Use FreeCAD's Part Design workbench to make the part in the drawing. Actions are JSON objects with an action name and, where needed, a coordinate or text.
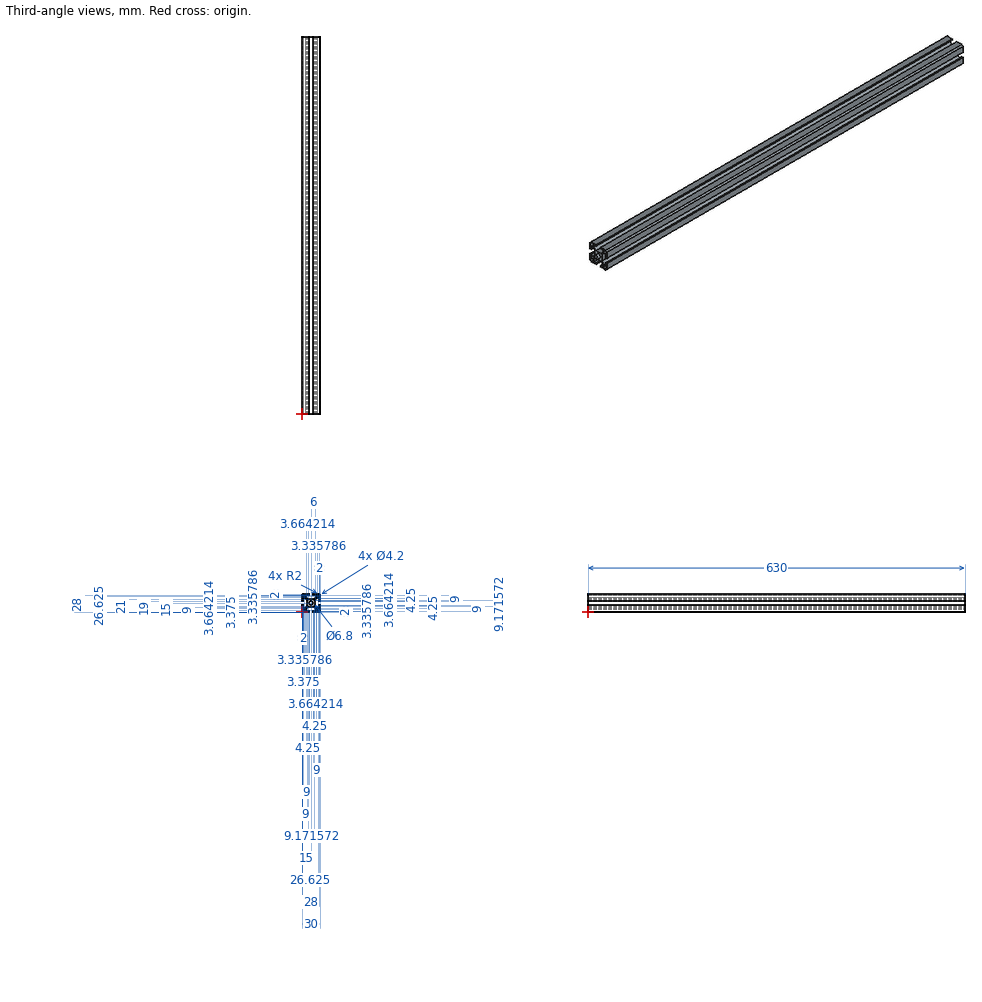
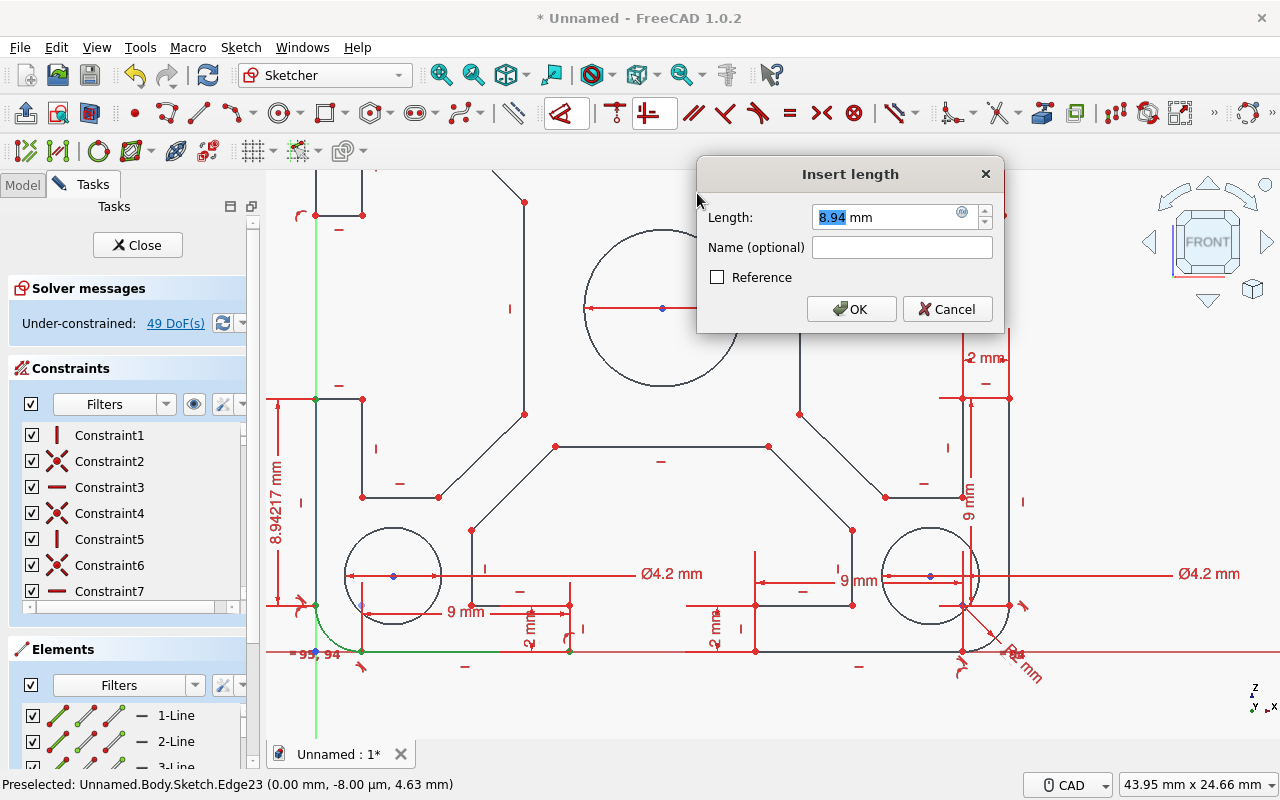
{"action": "type", "text": "9"}
{"action": "key", "text": "Return"}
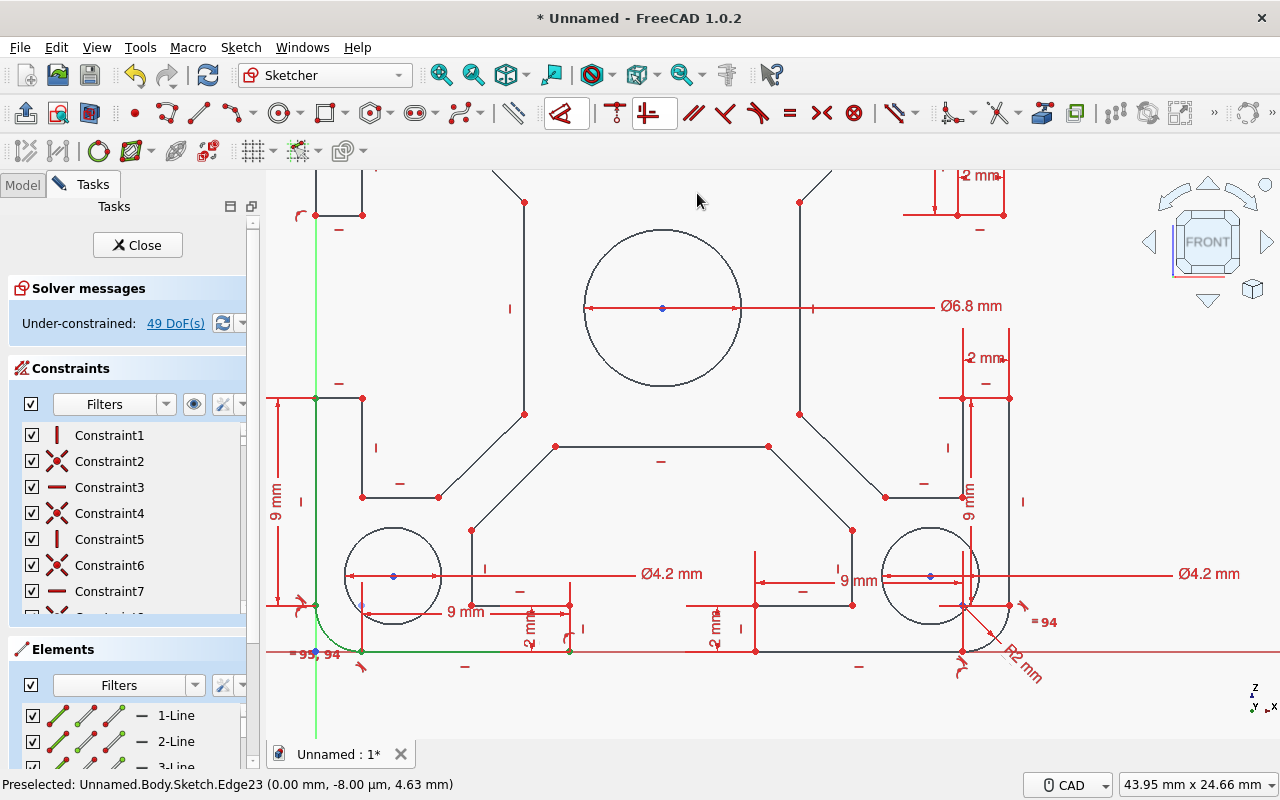
{"action": "left_click", "coordinate": [330, 398]}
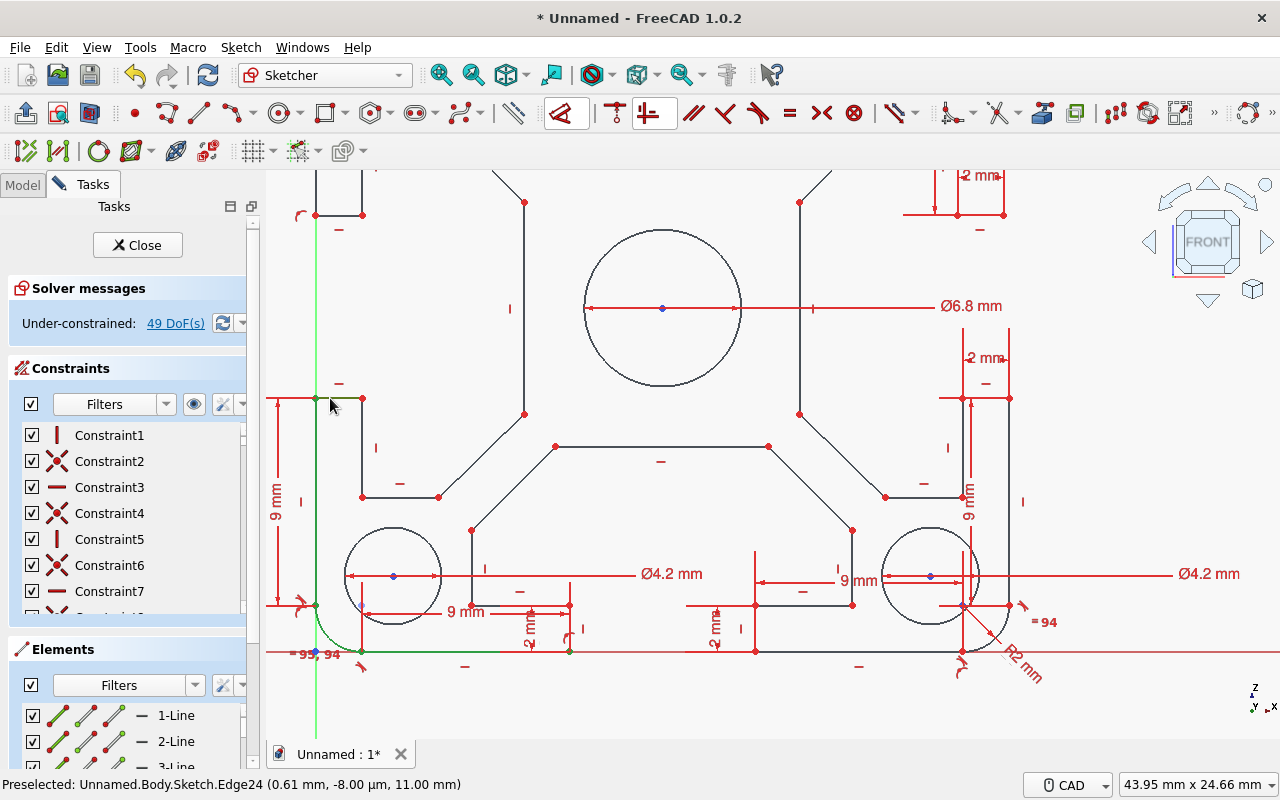
{"action": "key", "text": "l"}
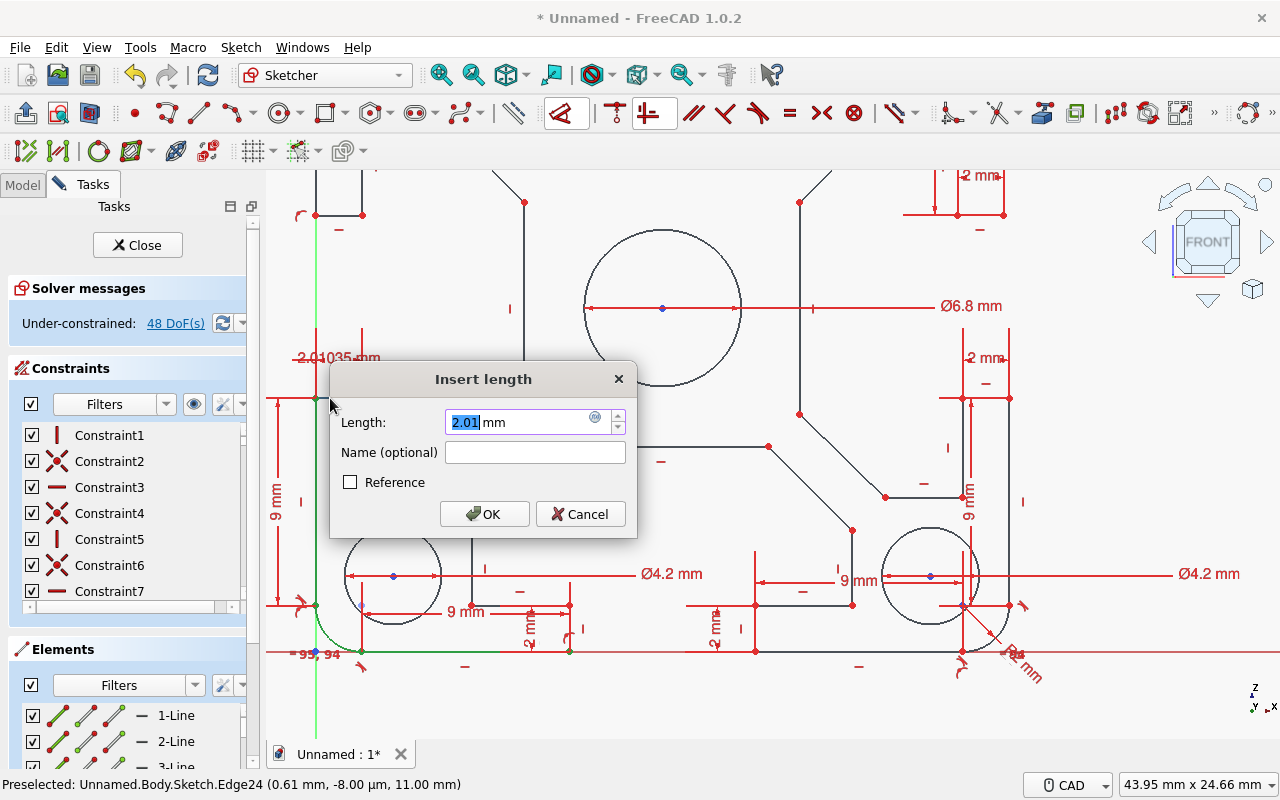
{"action": "type", "text": "2"}
{"action": "key", "text": "Return"}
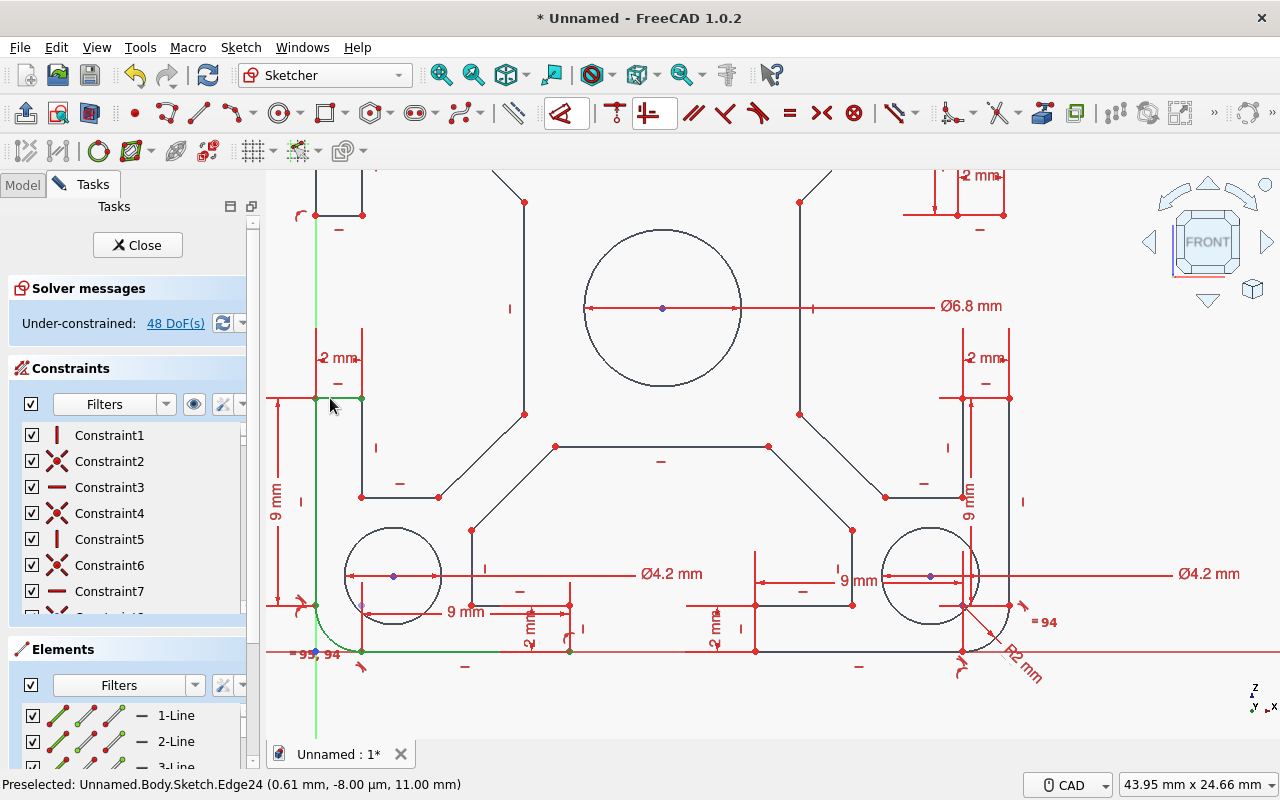
{"action": "left_click", "coordinate": [348, 216]}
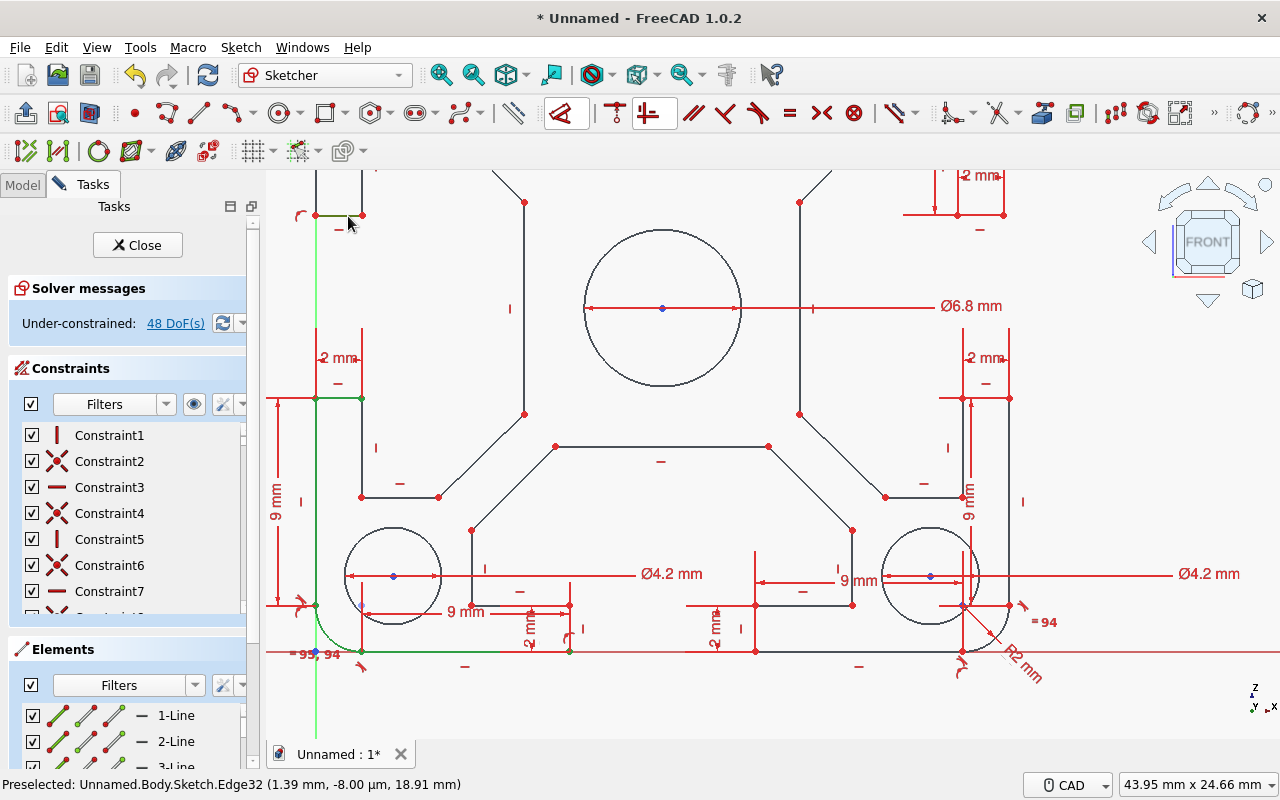
{"action": "left_click", "coordinate": [584, 114]}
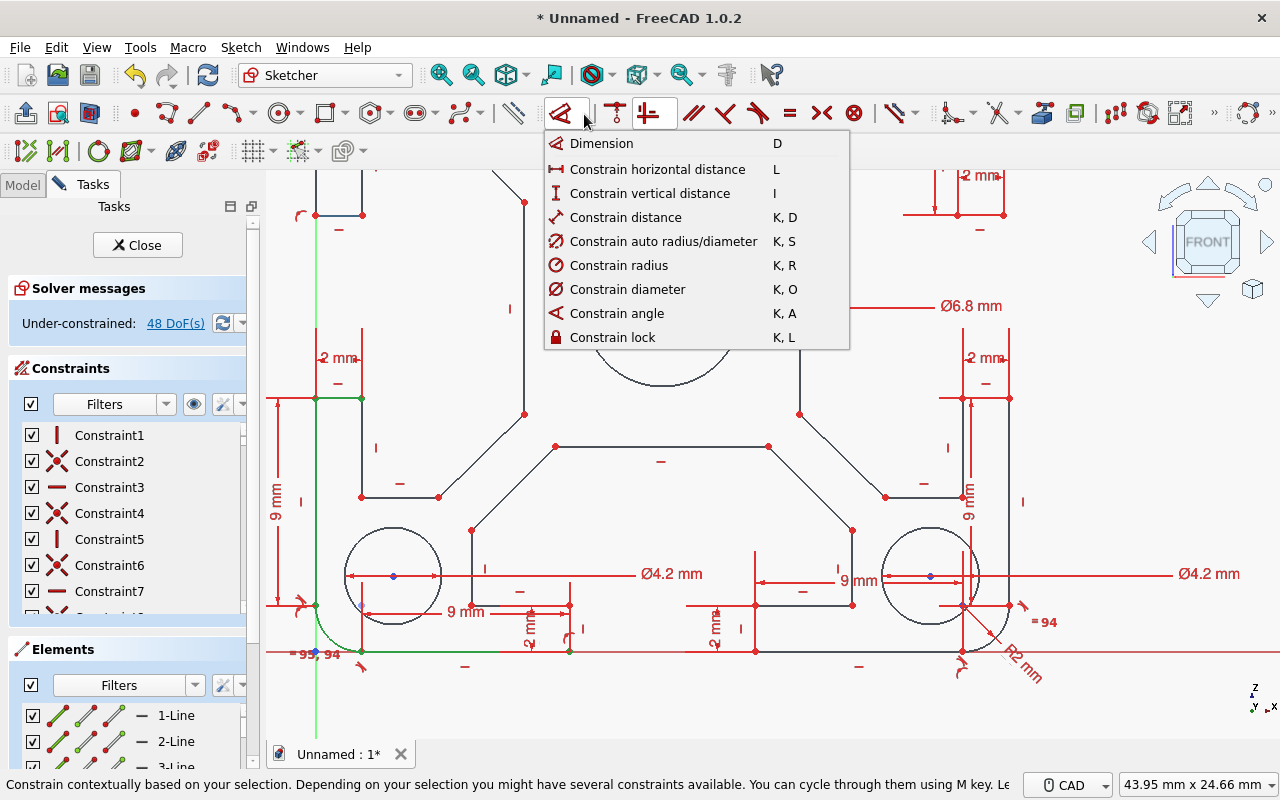
{"action": "left_click", "coordinate": [697, 169]}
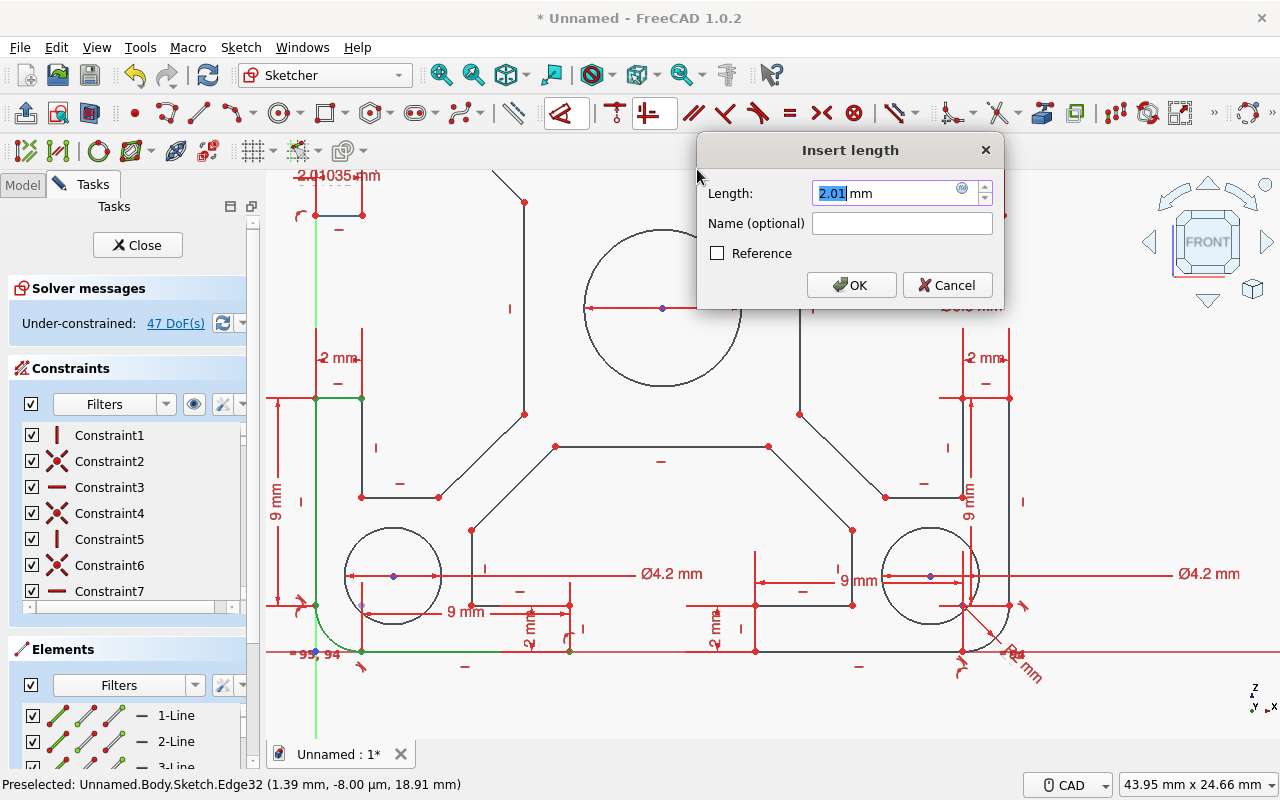
{"action": "type", "text": "2"}
{"action": "key", "text": "Return"}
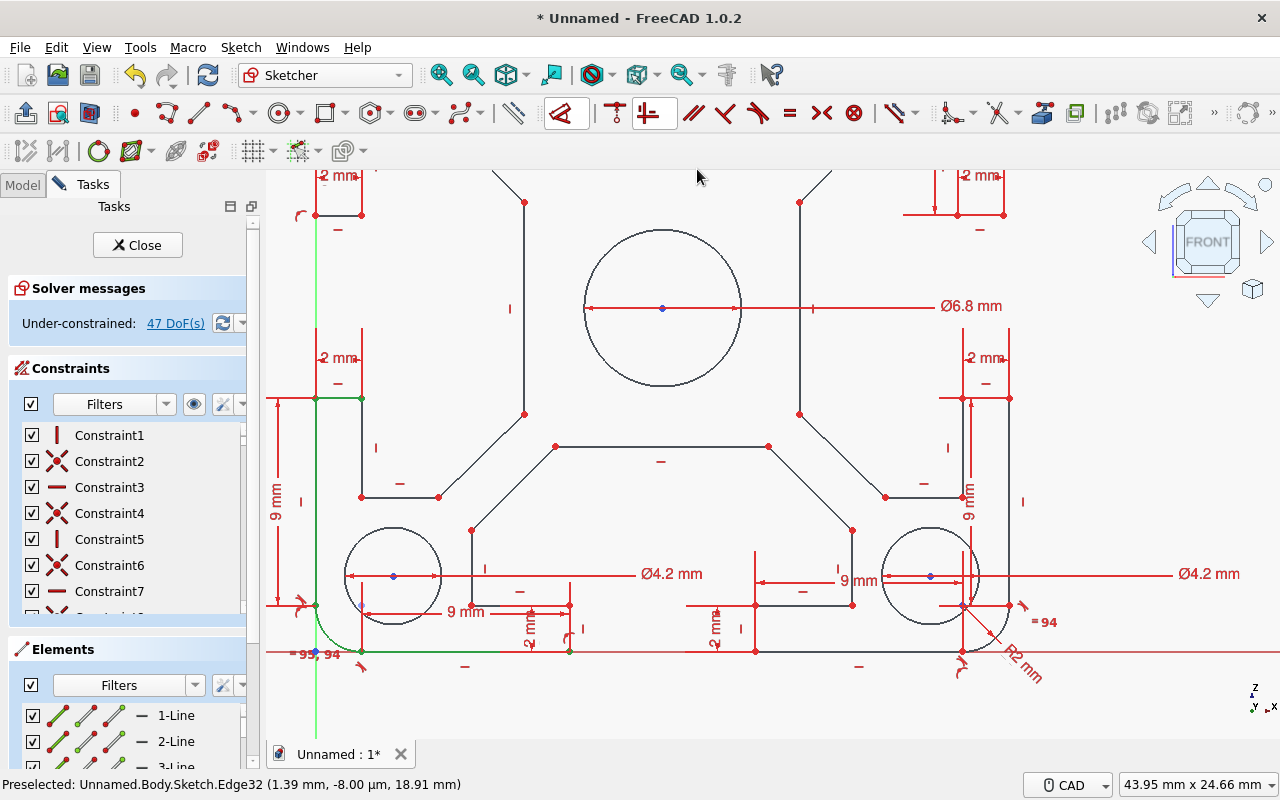
{"action": "scroll", "coordinate": [756, 635], "scroll_direction": "down", "scroll_amount": 3}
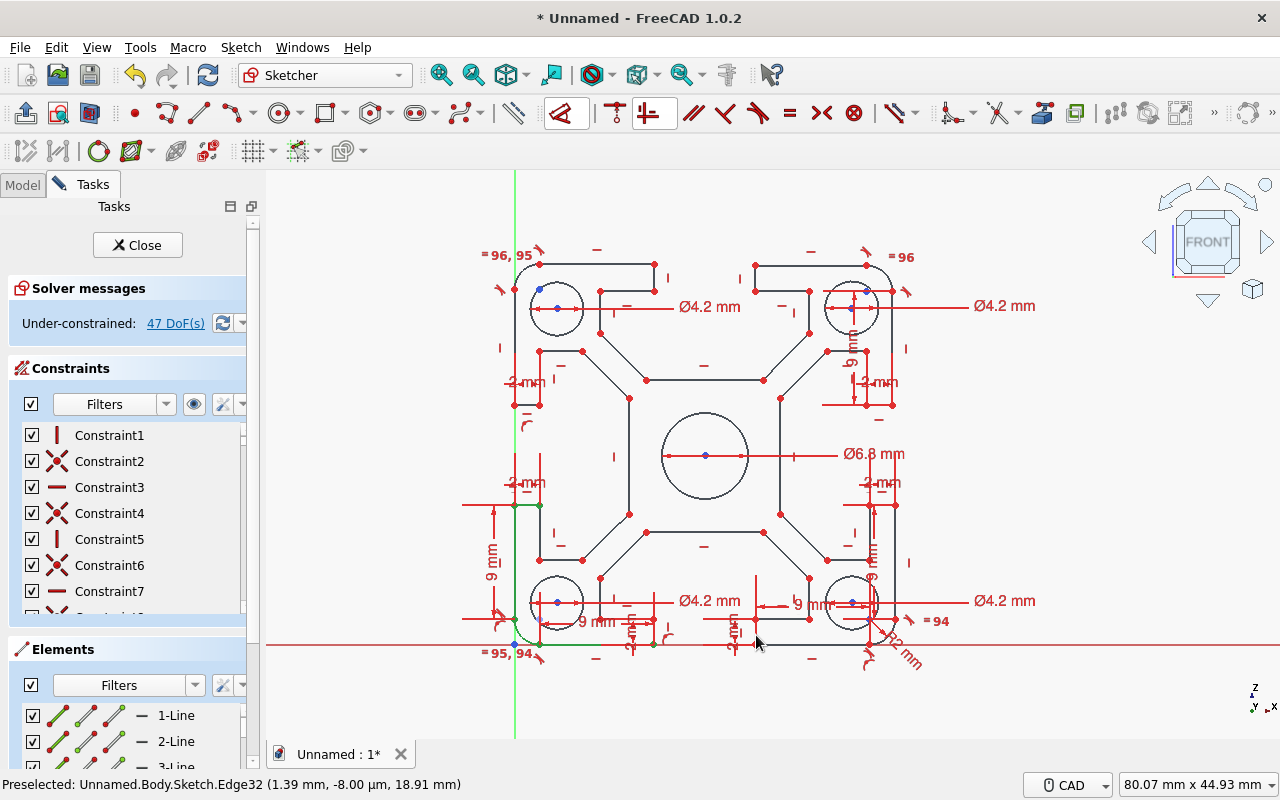
{"action": "left_click", "coordinate": [515, 370]}